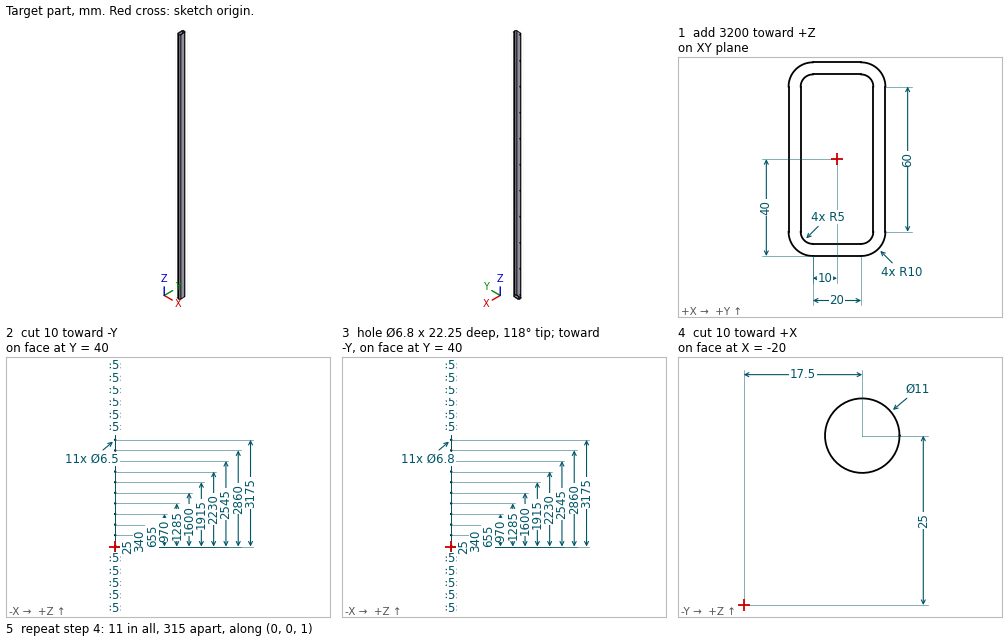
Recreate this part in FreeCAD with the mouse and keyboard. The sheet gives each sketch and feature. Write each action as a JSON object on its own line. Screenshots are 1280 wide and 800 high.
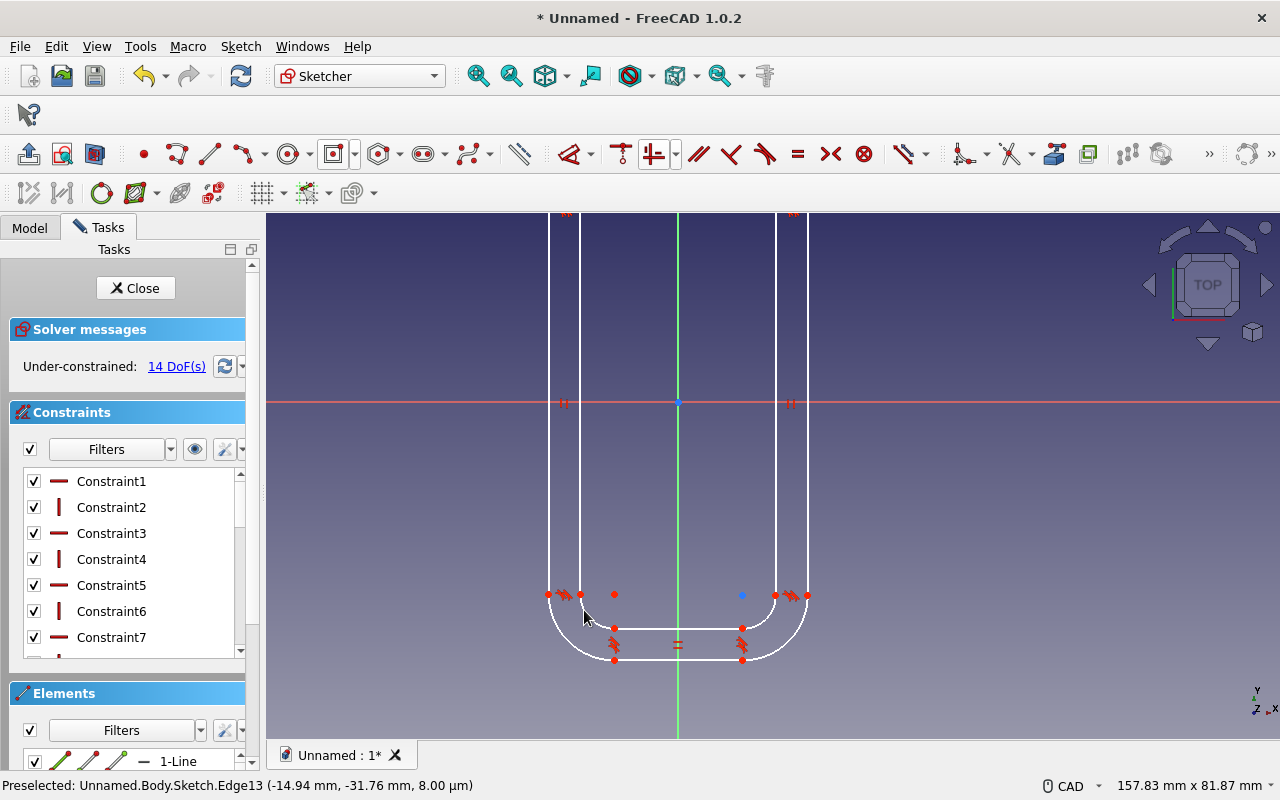
{"action": "scroll", "coordinate": [757, 626], "scroll_direction": "down", "scroll_amount": 2}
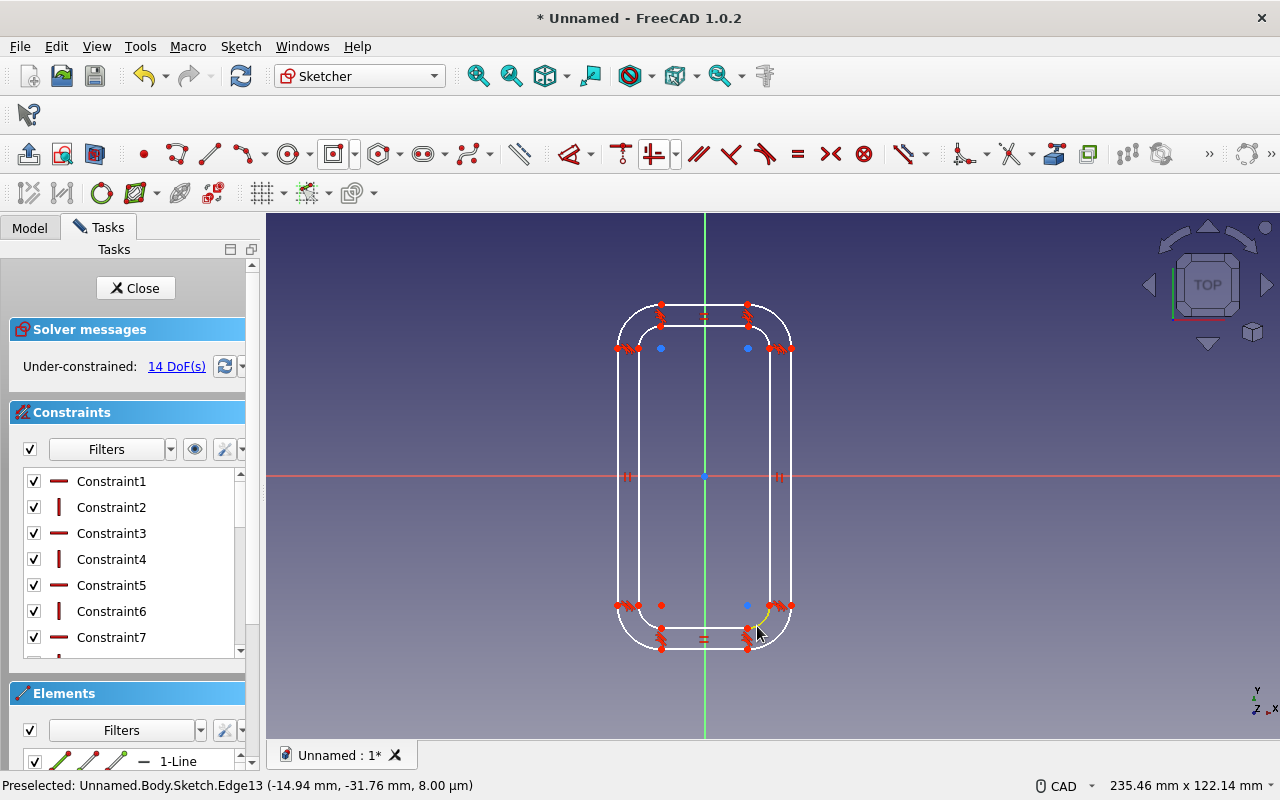
{"action": "left_click", "coordinate": [641, 310]}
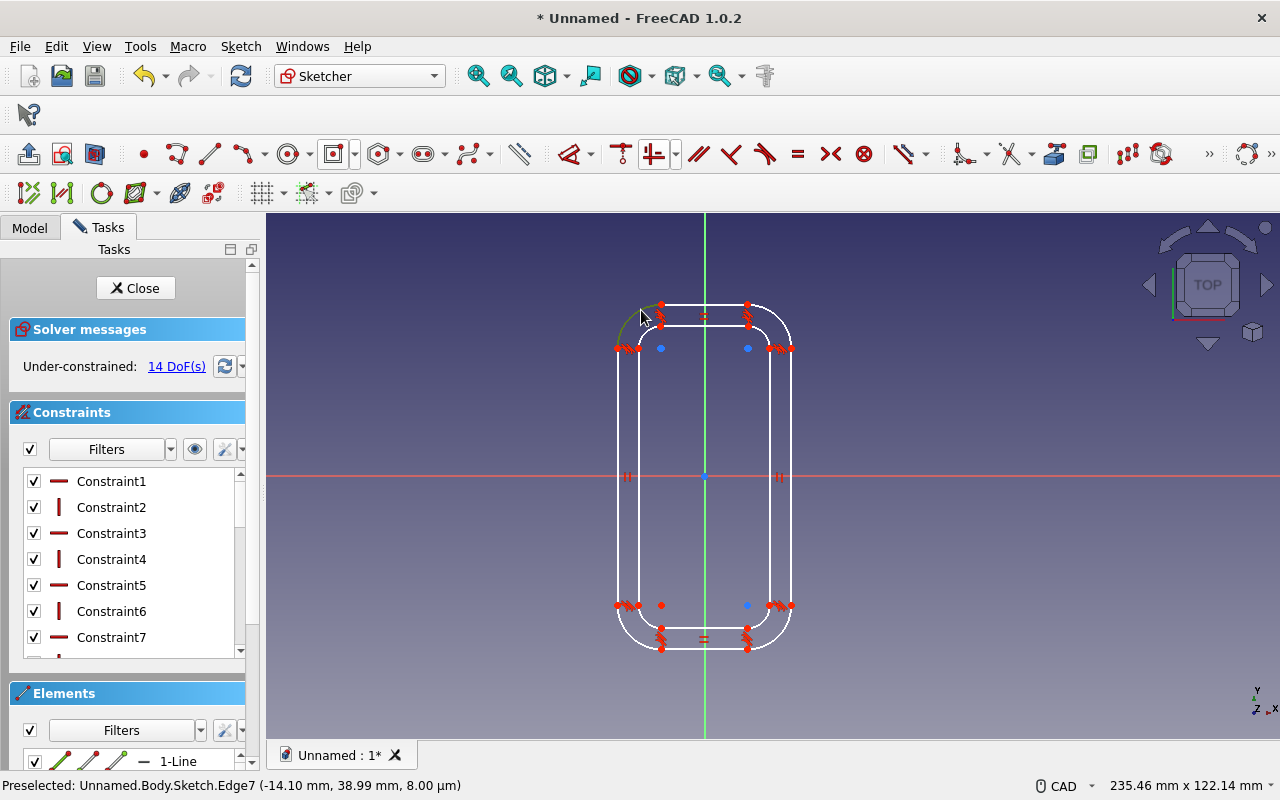
{"action": "scroll", "coordinate": [651, 329], "scroll_direction": "up", "scroll_amount": 2}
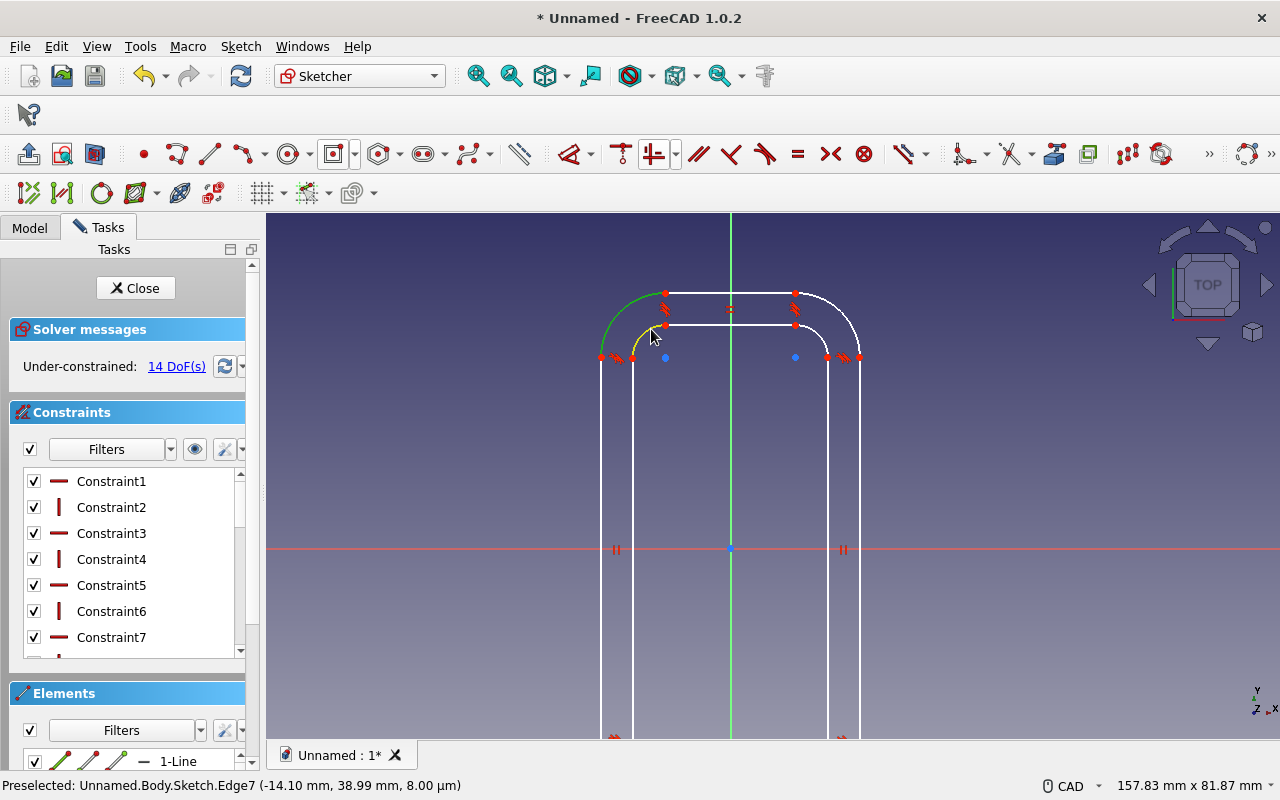
{"action": "left_click", "coordinate": [651, 329]}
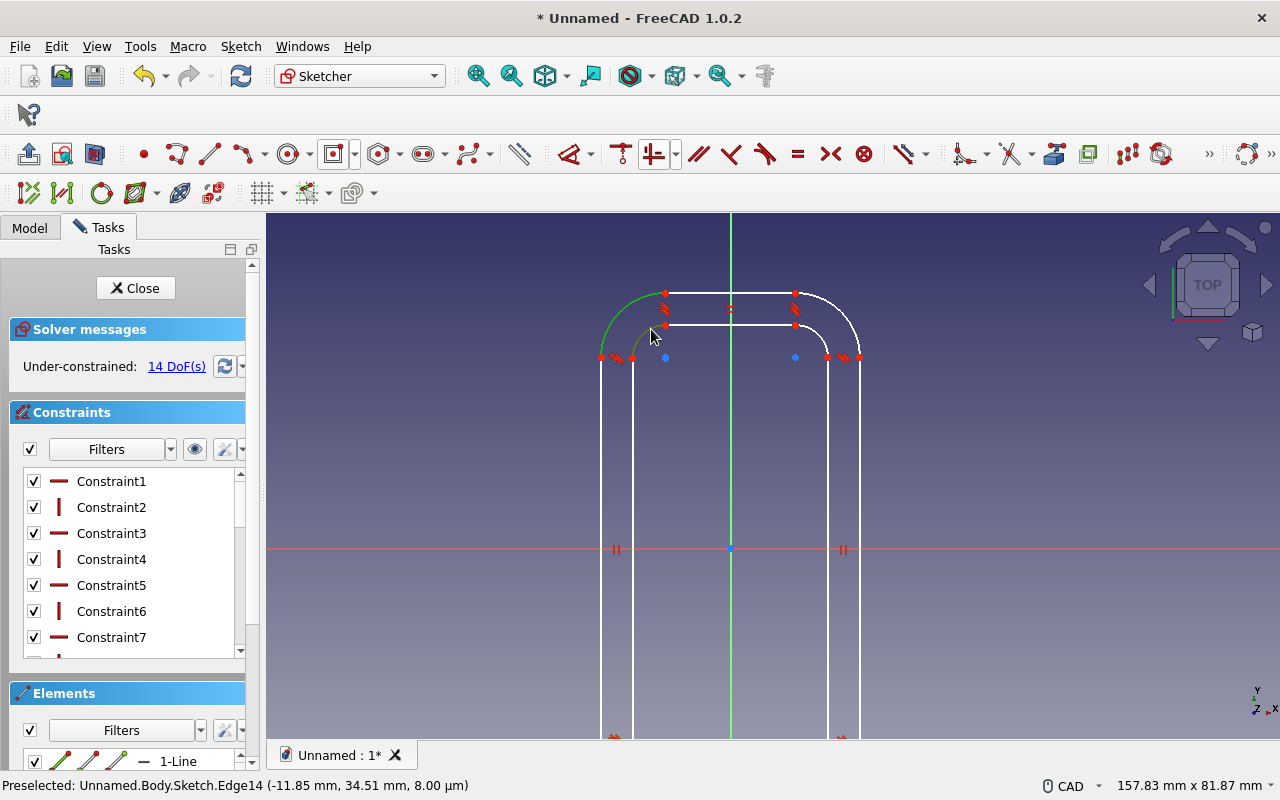
{"action": "left_click", "coordinate": [621, 154]}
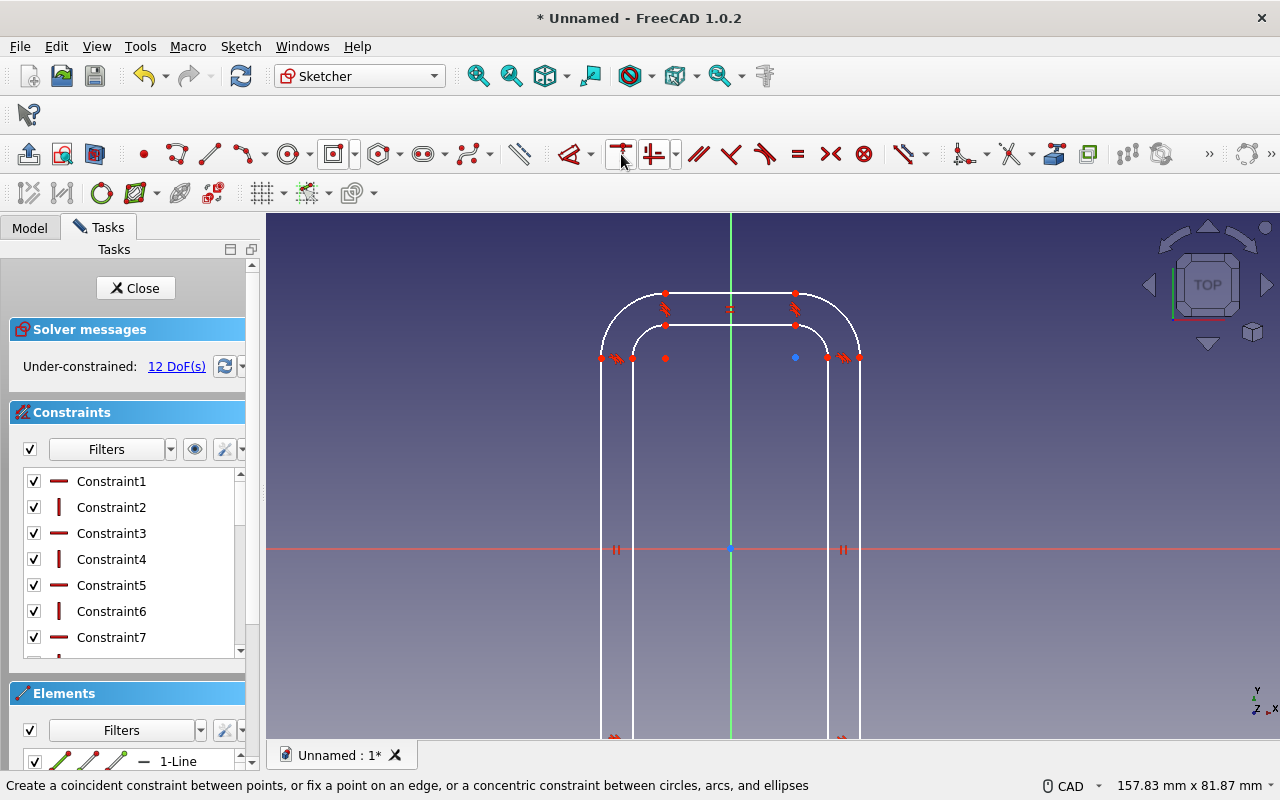
{"action": "left_click", "coordinate": [853, 328]}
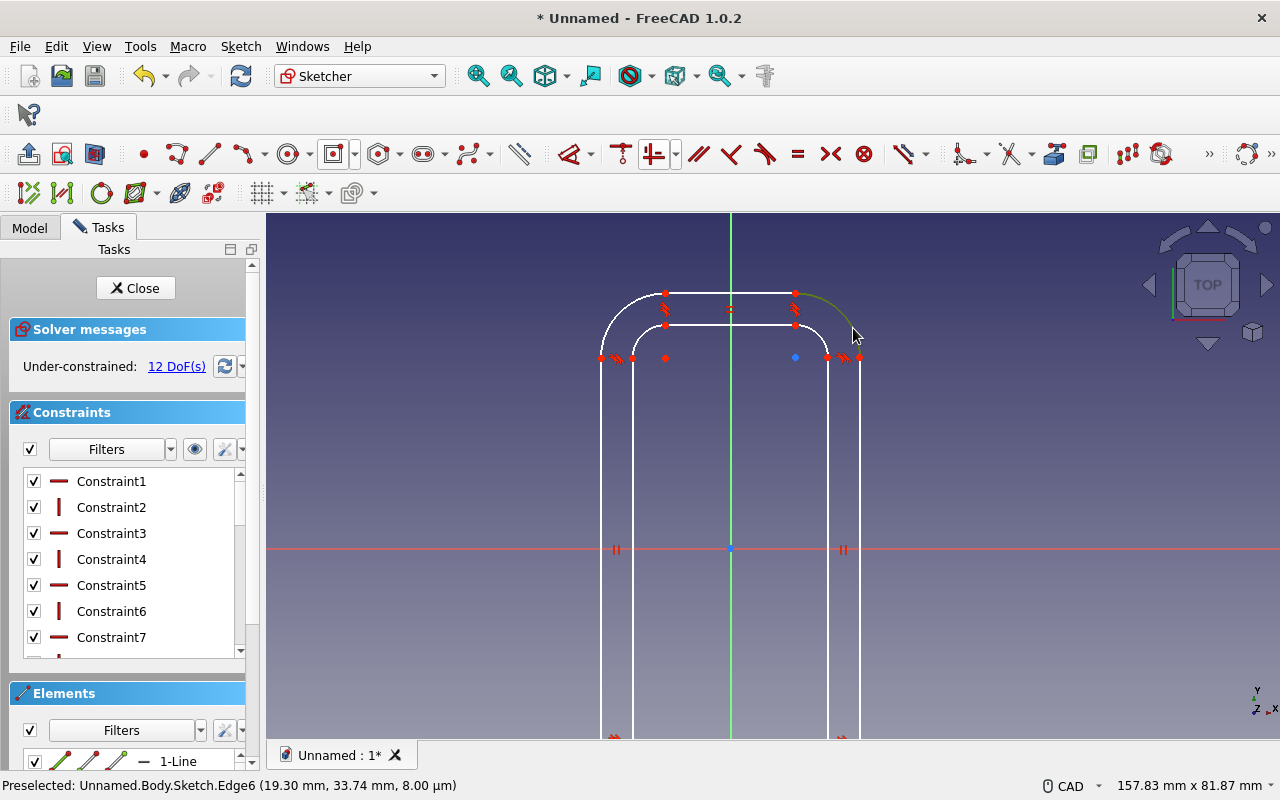
{"action": "left_click", "coordinate": [824, 343]}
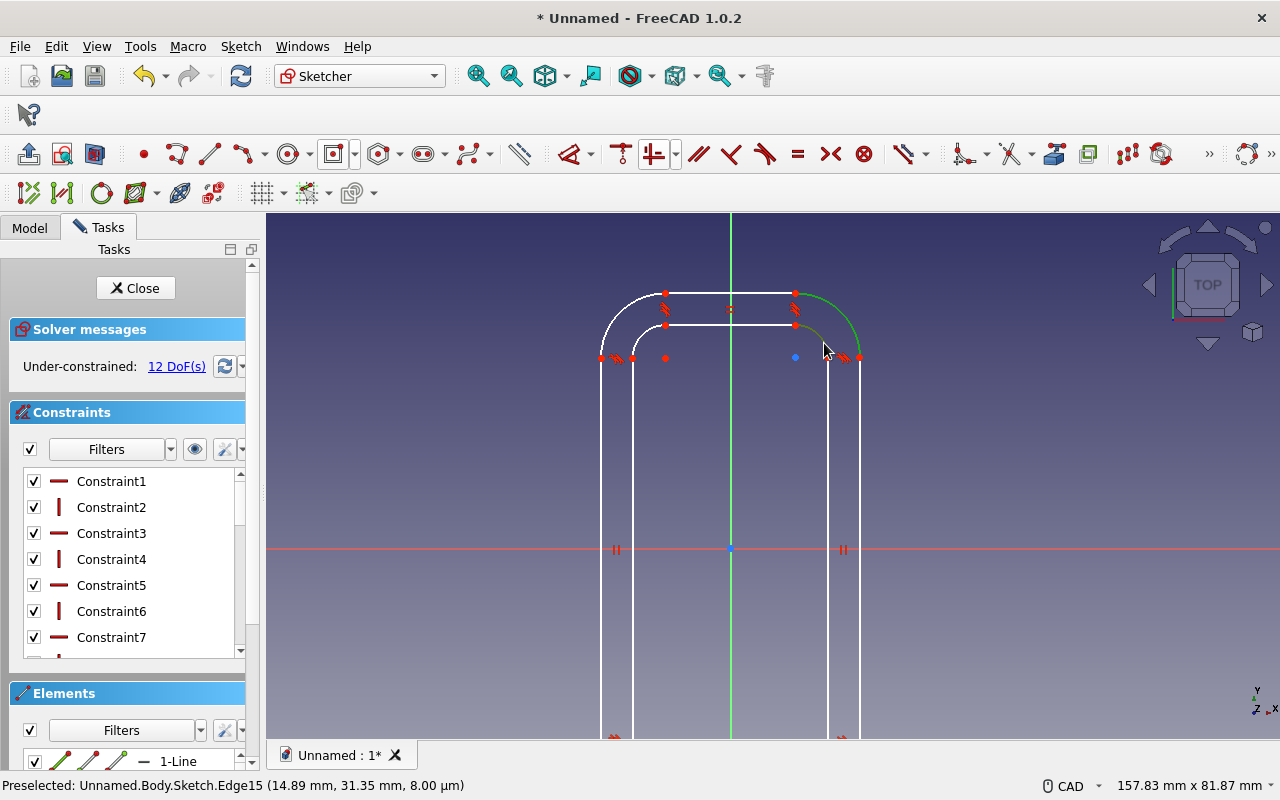
{"action": "left_click", "coordinate": [621, 154]}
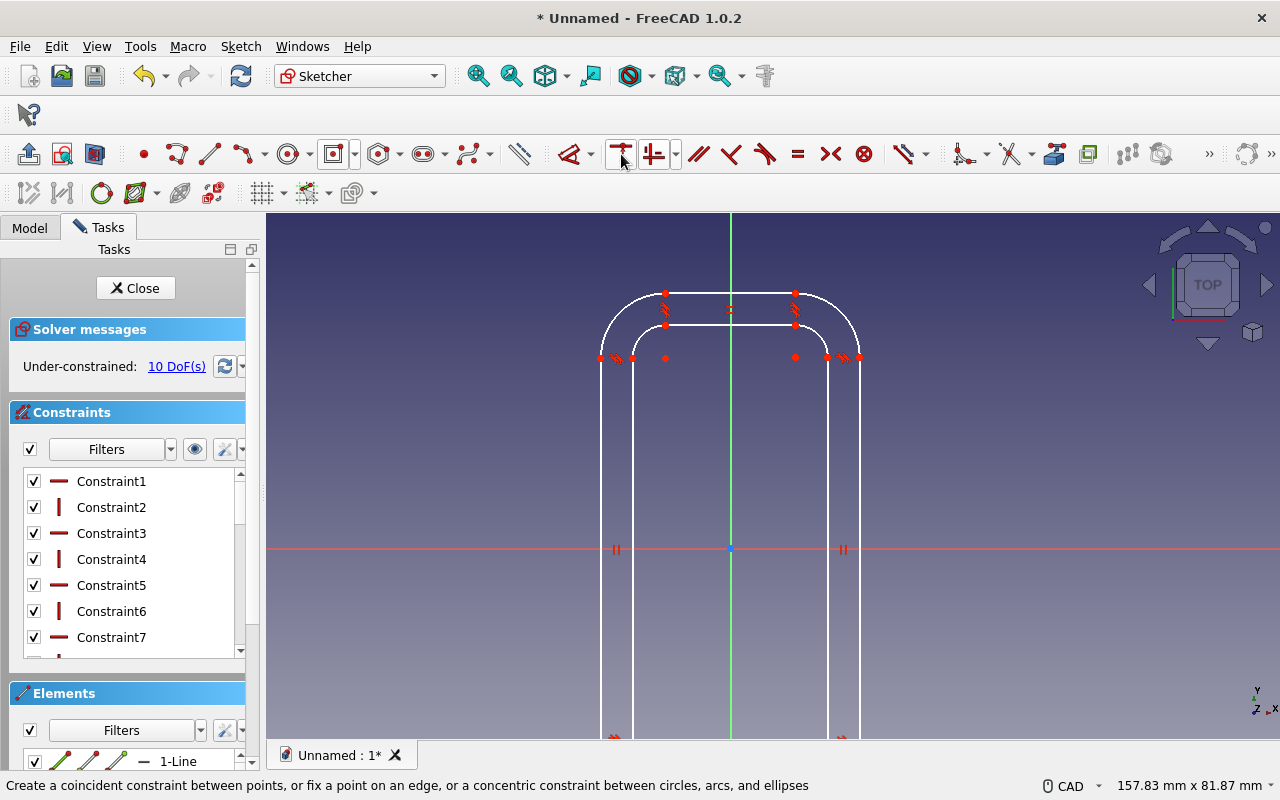
{"action": "scroll", "coordinate": [651, 328], "scroll_direction": "down", "scroll_amount": 2}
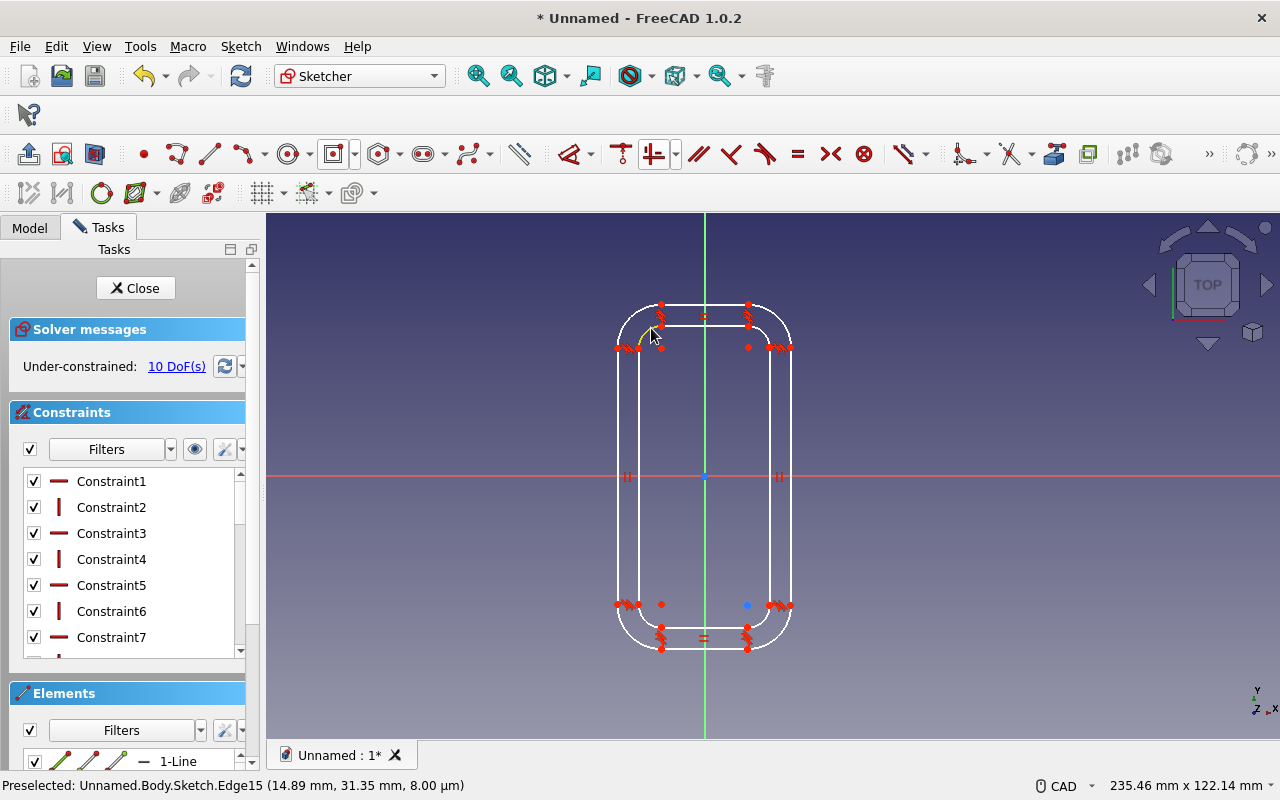
{"action": "left_click", "coordinate": [767, 644]}